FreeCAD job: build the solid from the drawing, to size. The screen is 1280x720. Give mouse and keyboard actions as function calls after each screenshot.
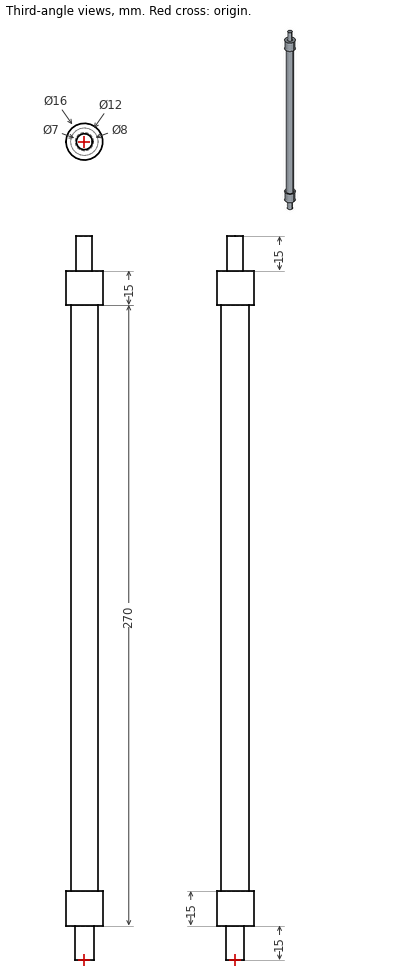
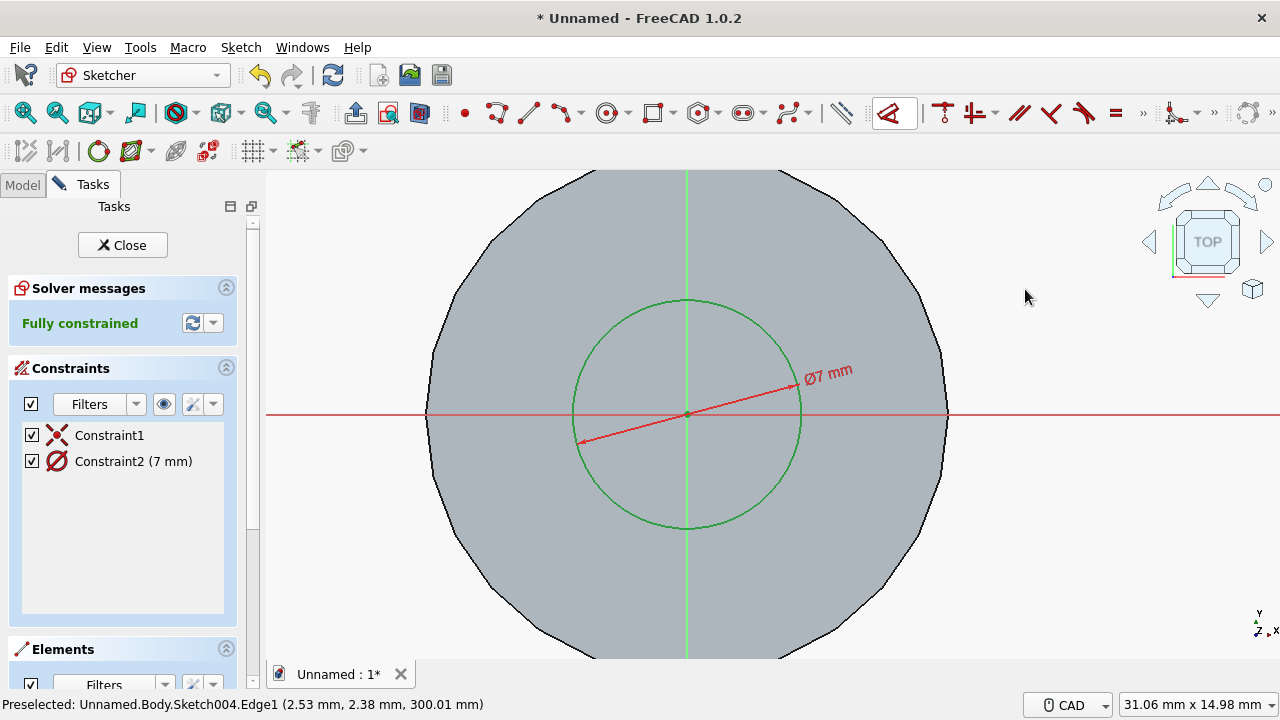
click(123, 245)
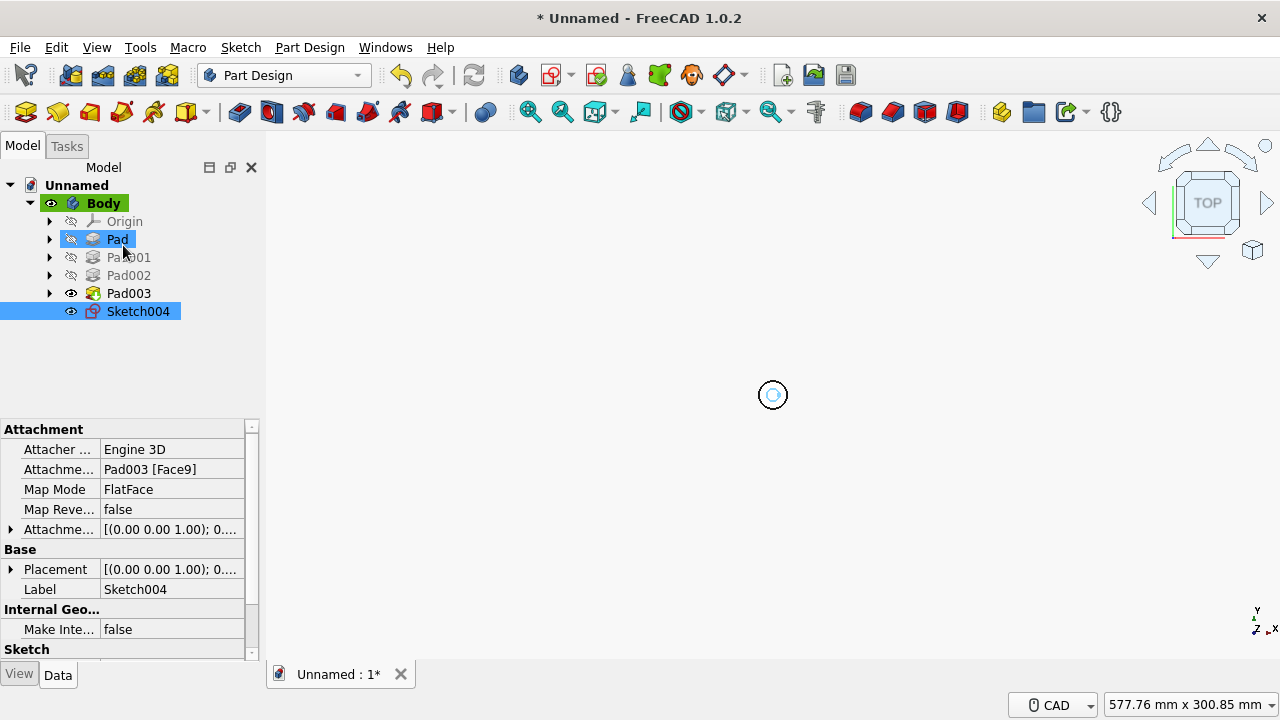
click(26, 112)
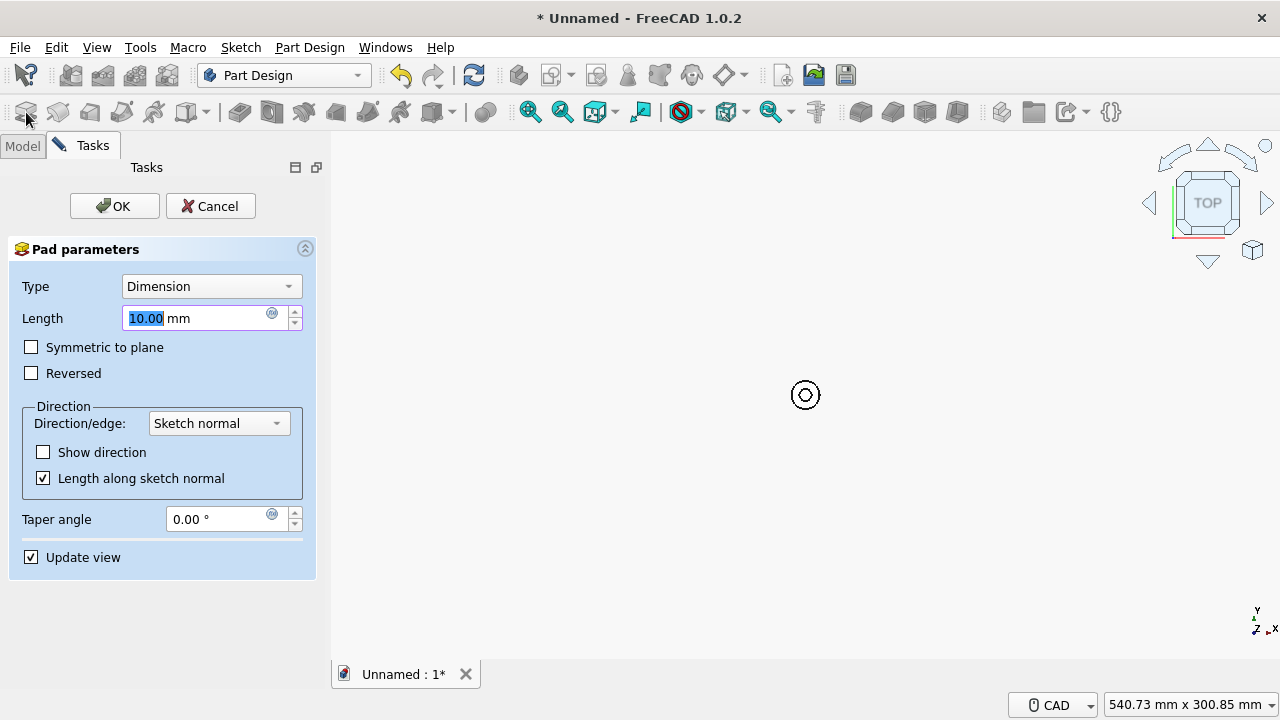
text(15)
key(Tab)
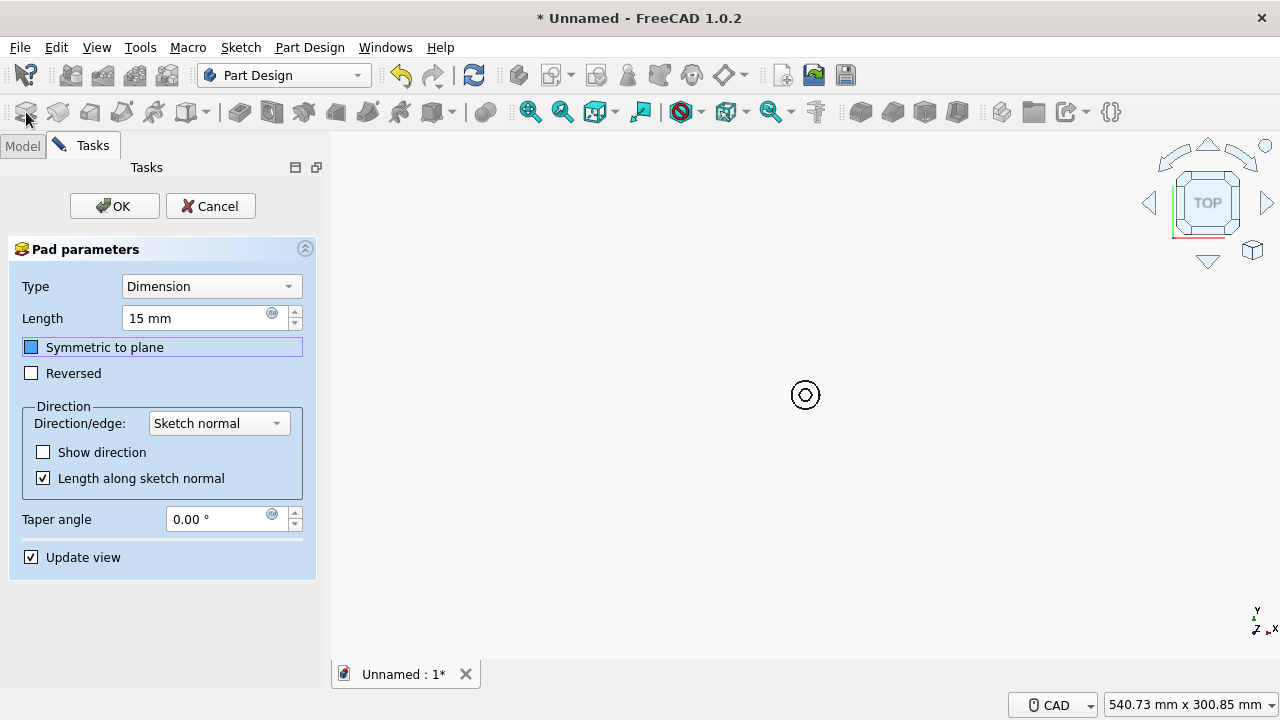
click(115, 206)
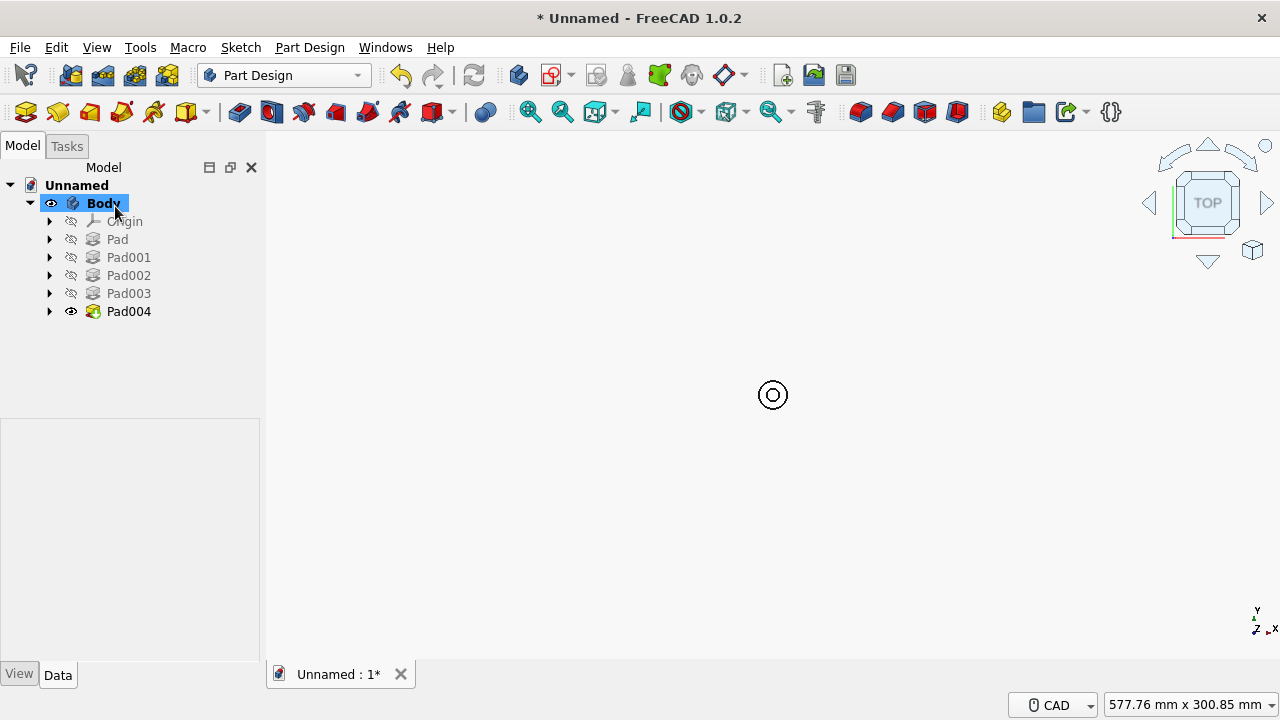
key(0)